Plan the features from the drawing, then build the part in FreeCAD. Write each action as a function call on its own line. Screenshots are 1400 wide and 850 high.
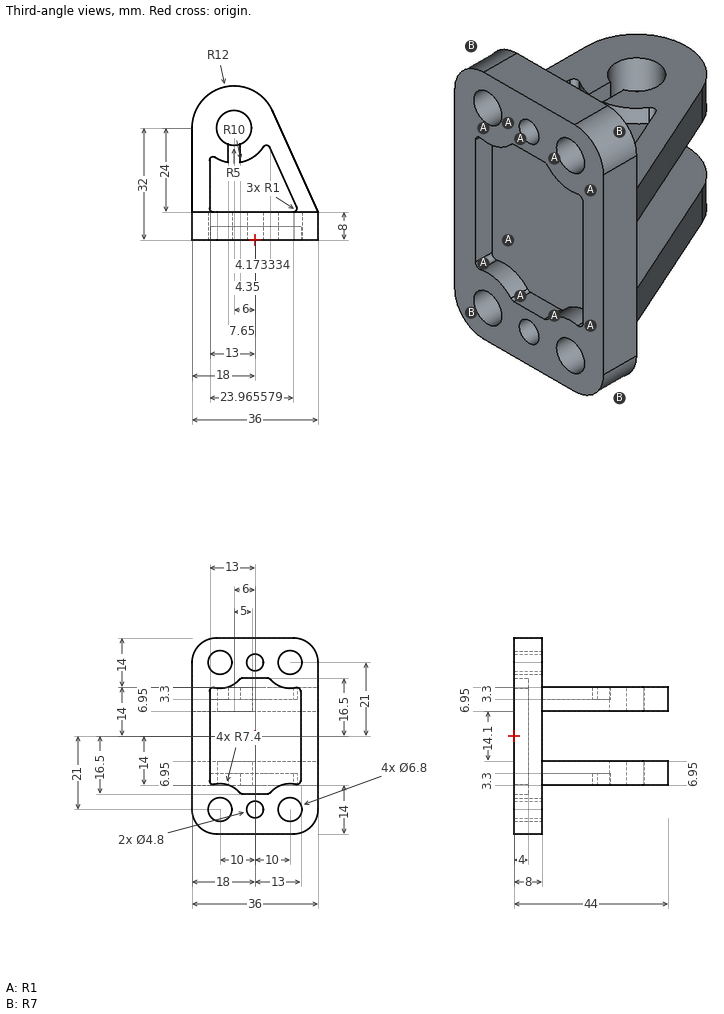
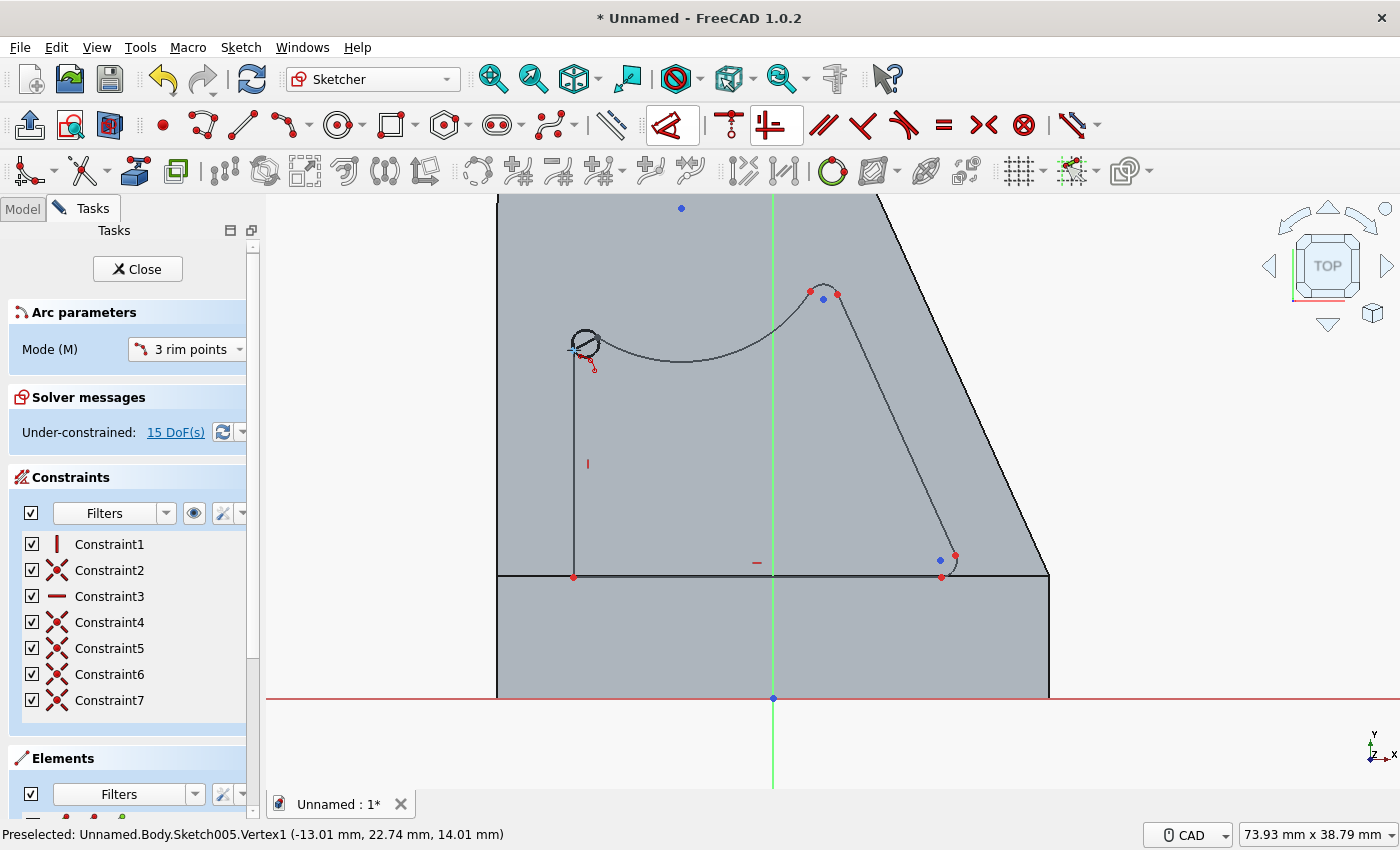
scroll(582, 336, up, 4)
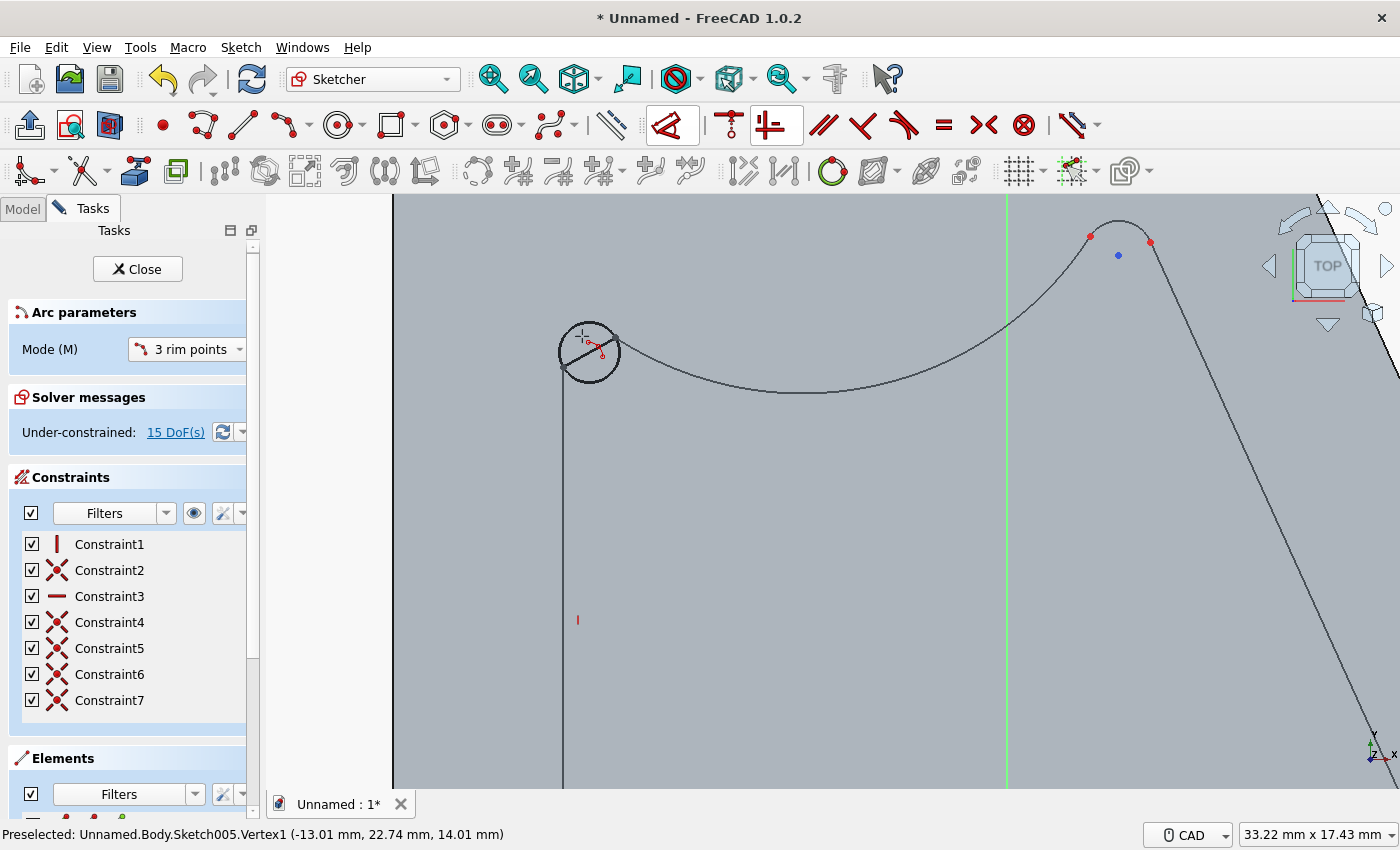
click(581, 336)
key(Escape)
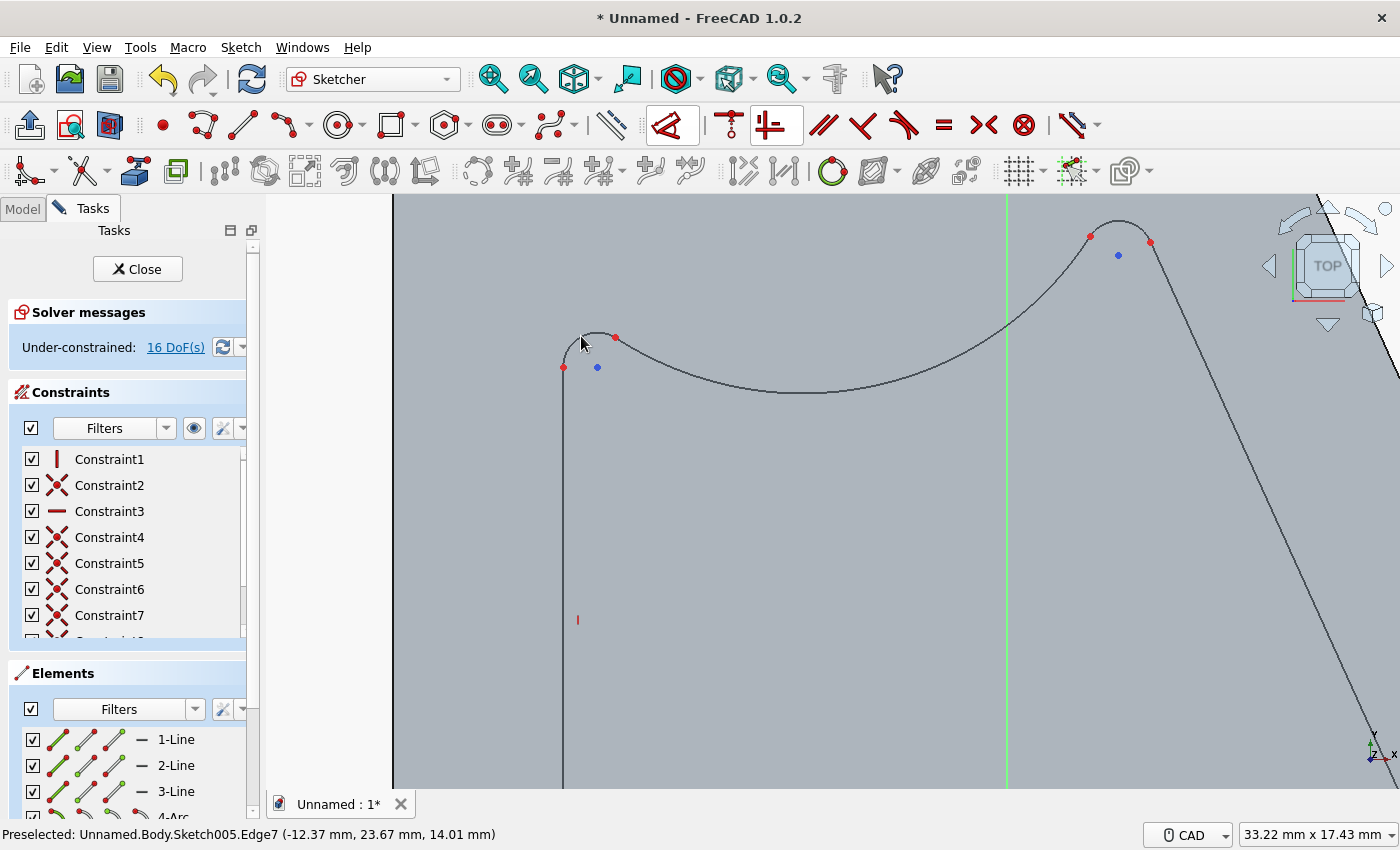
click(563, 519)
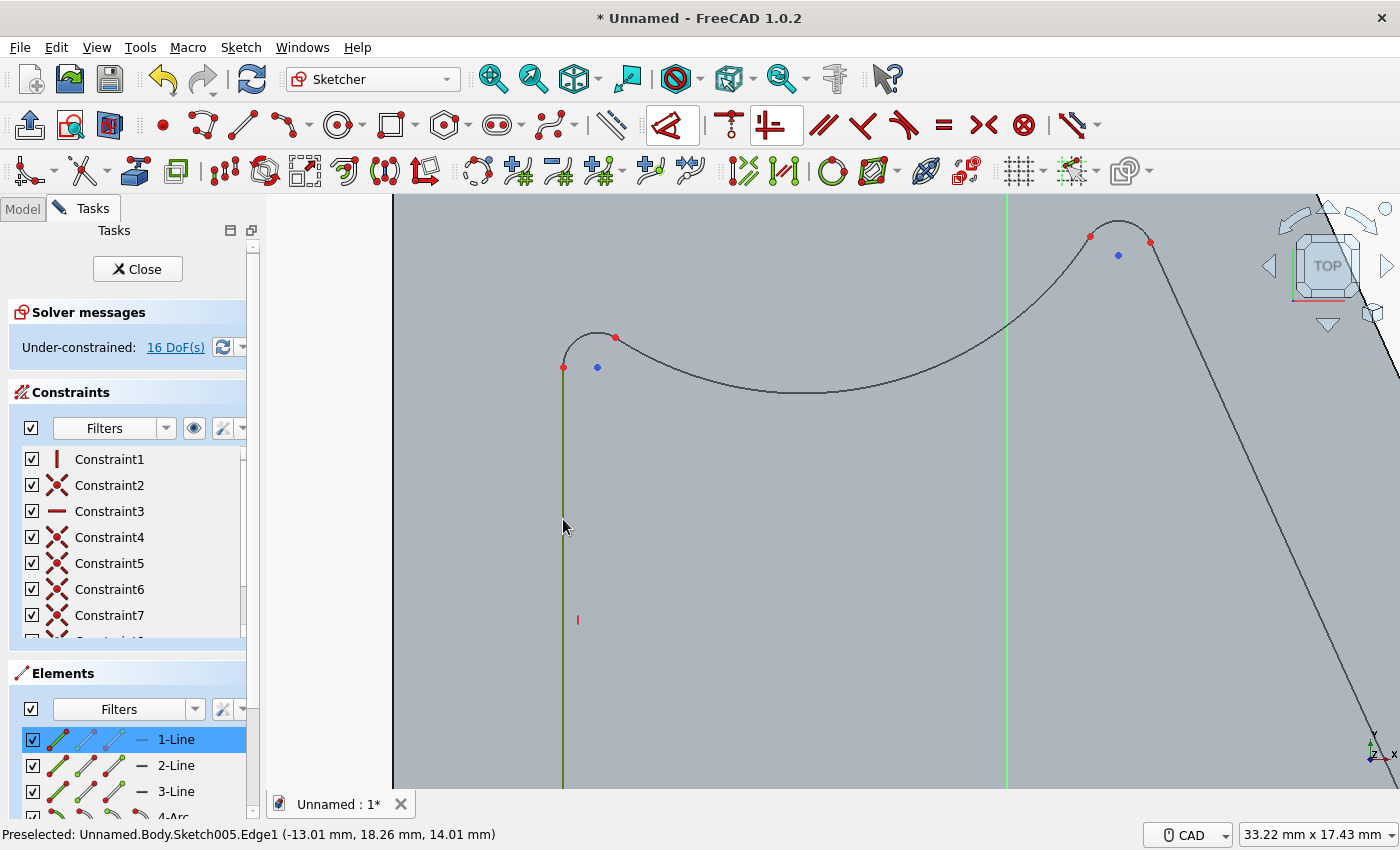
click(595, 333)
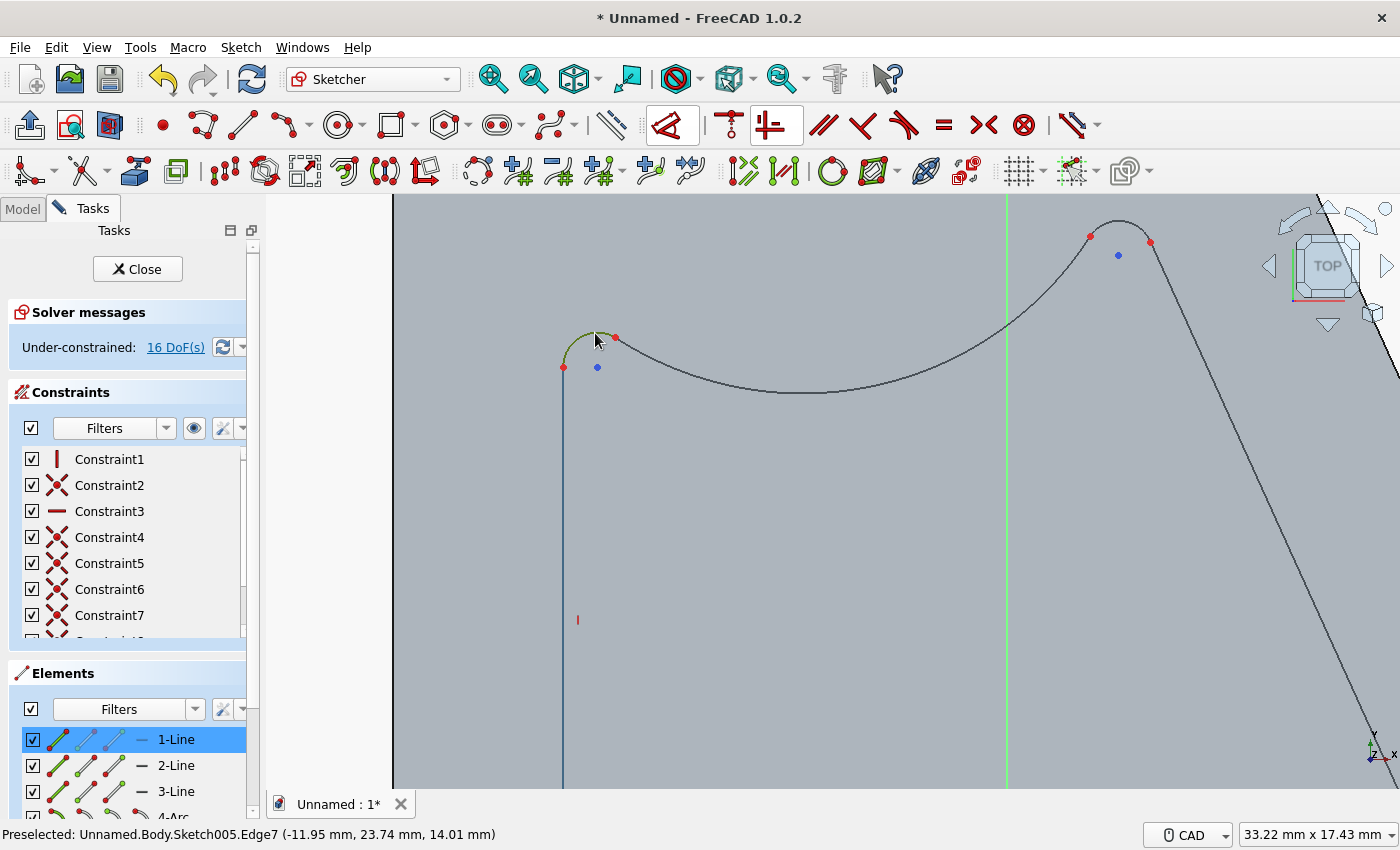
click(904, 126)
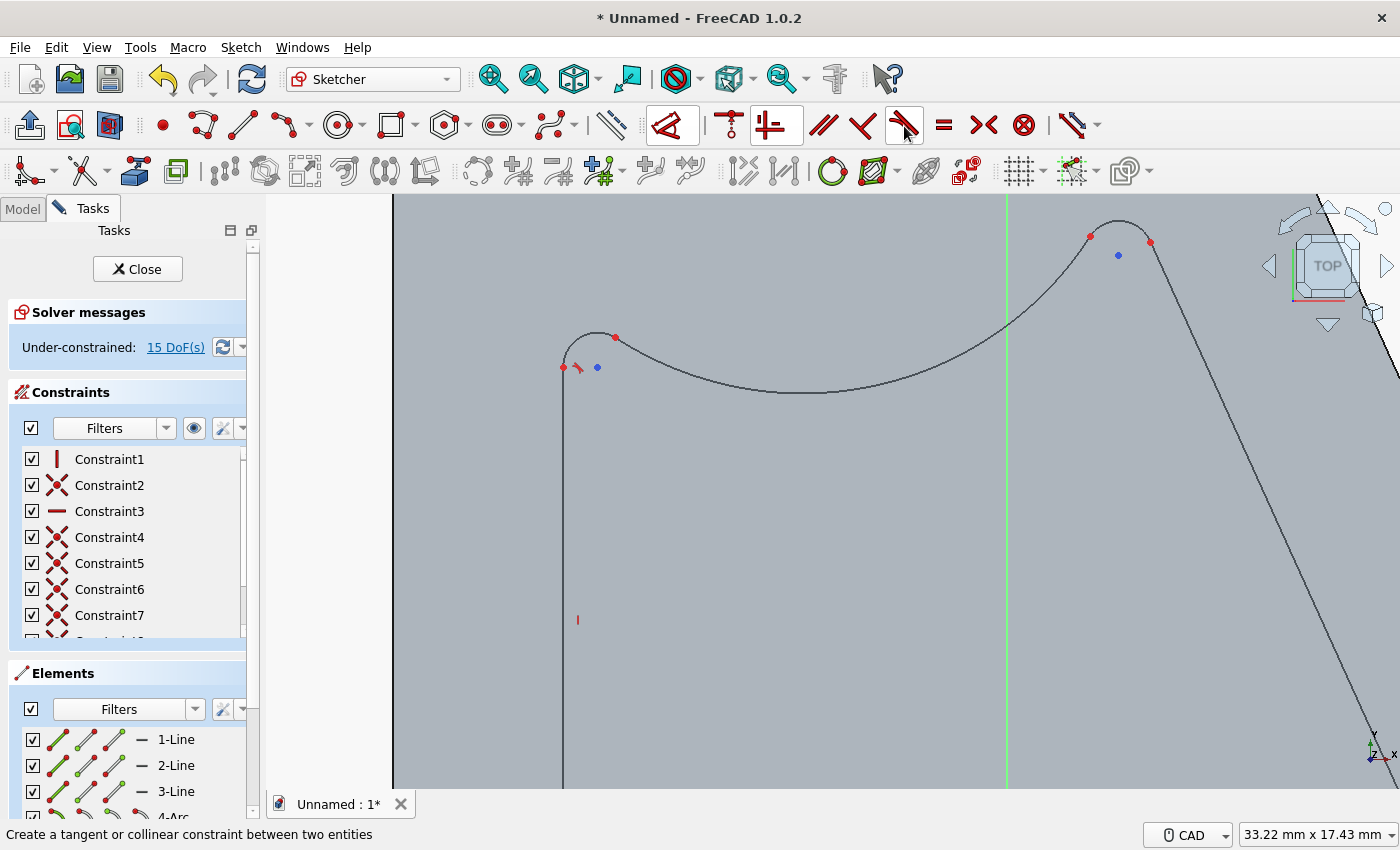
scroll(582, 337, down, 4)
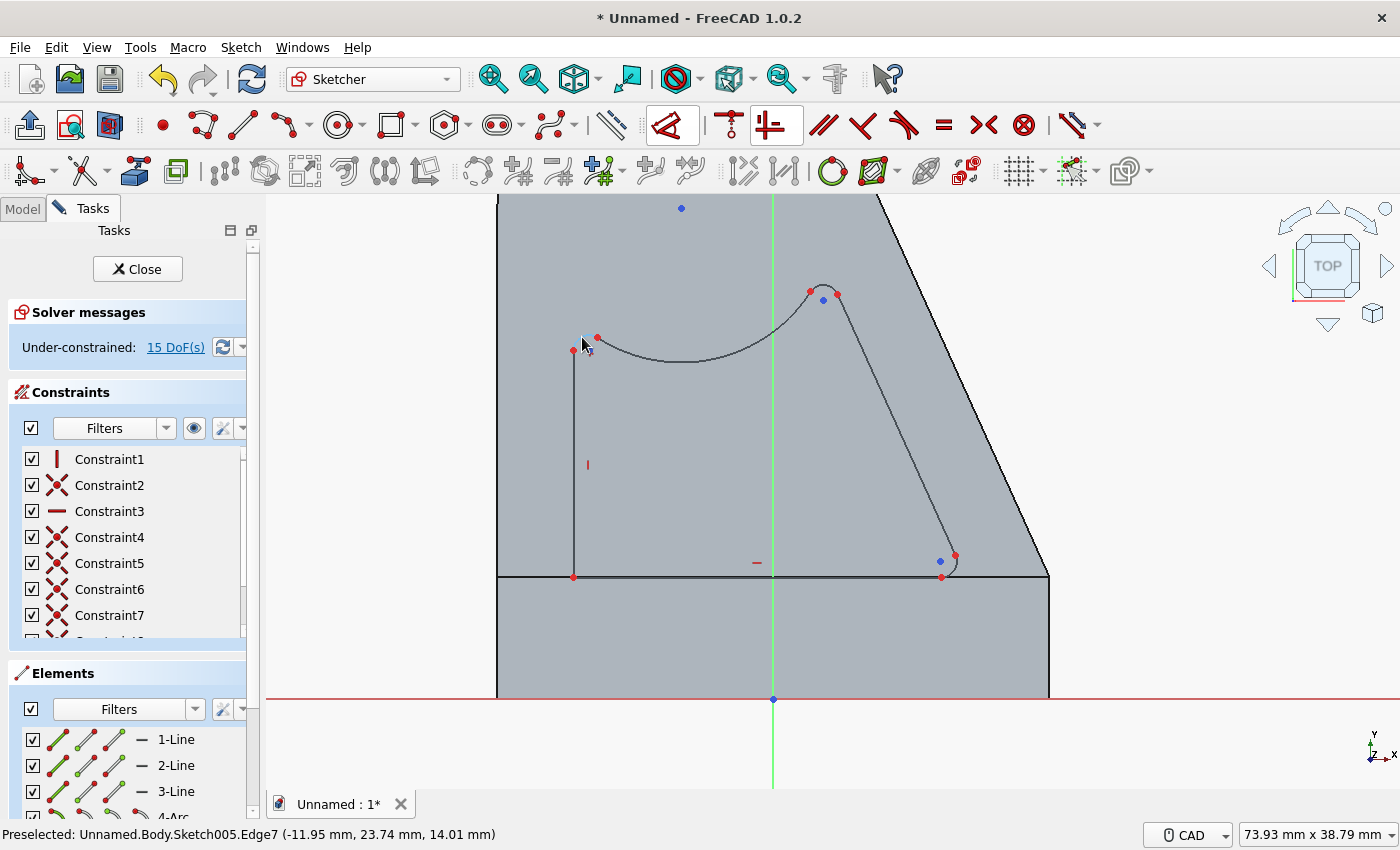
click(684, 578)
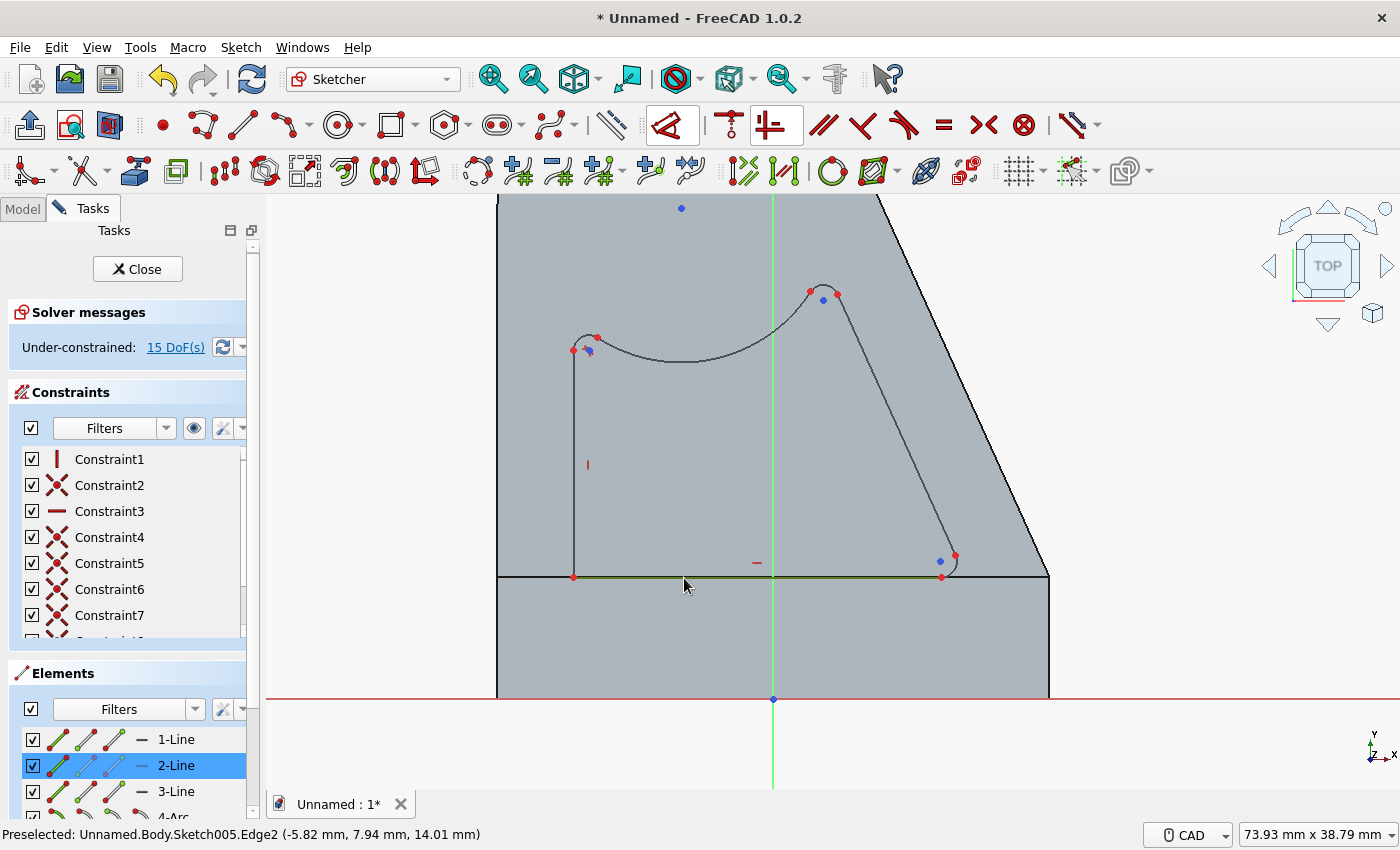
click(954, 570)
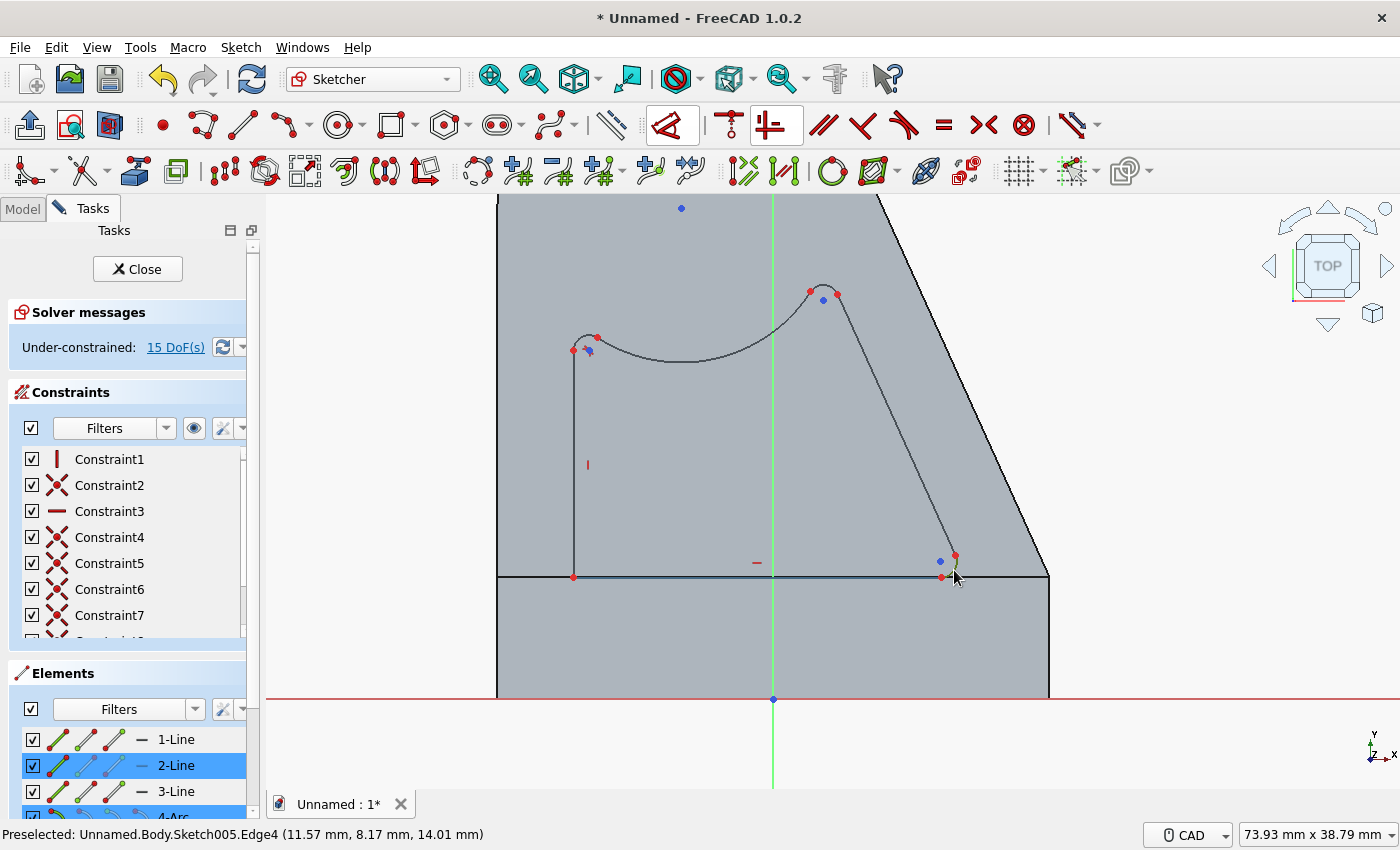
click(904, 126)